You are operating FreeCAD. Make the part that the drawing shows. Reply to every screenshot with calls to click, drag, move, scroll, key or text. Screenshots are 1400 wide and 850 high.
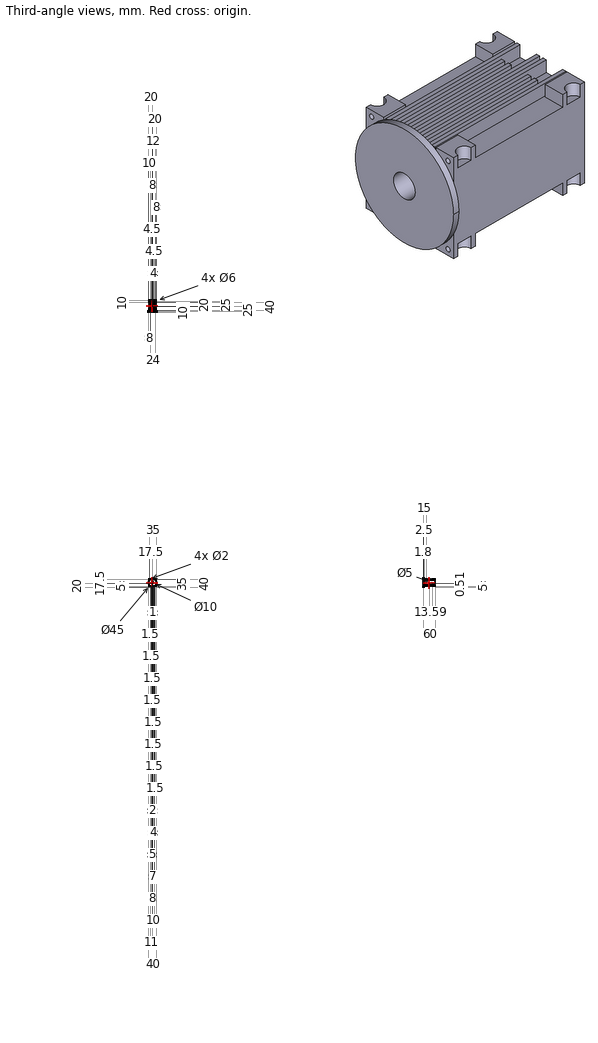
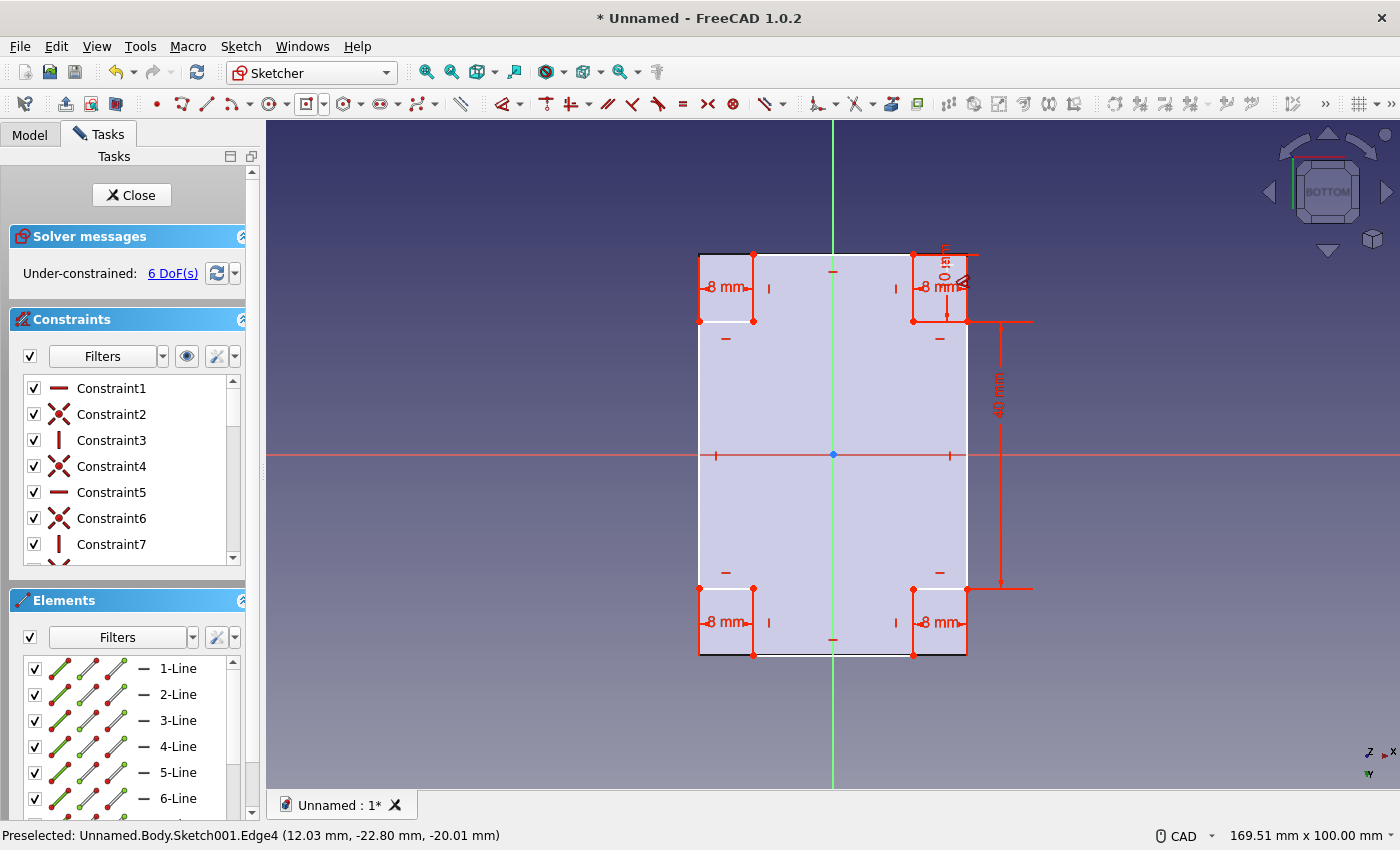
click(865, 255)
click(796, 221)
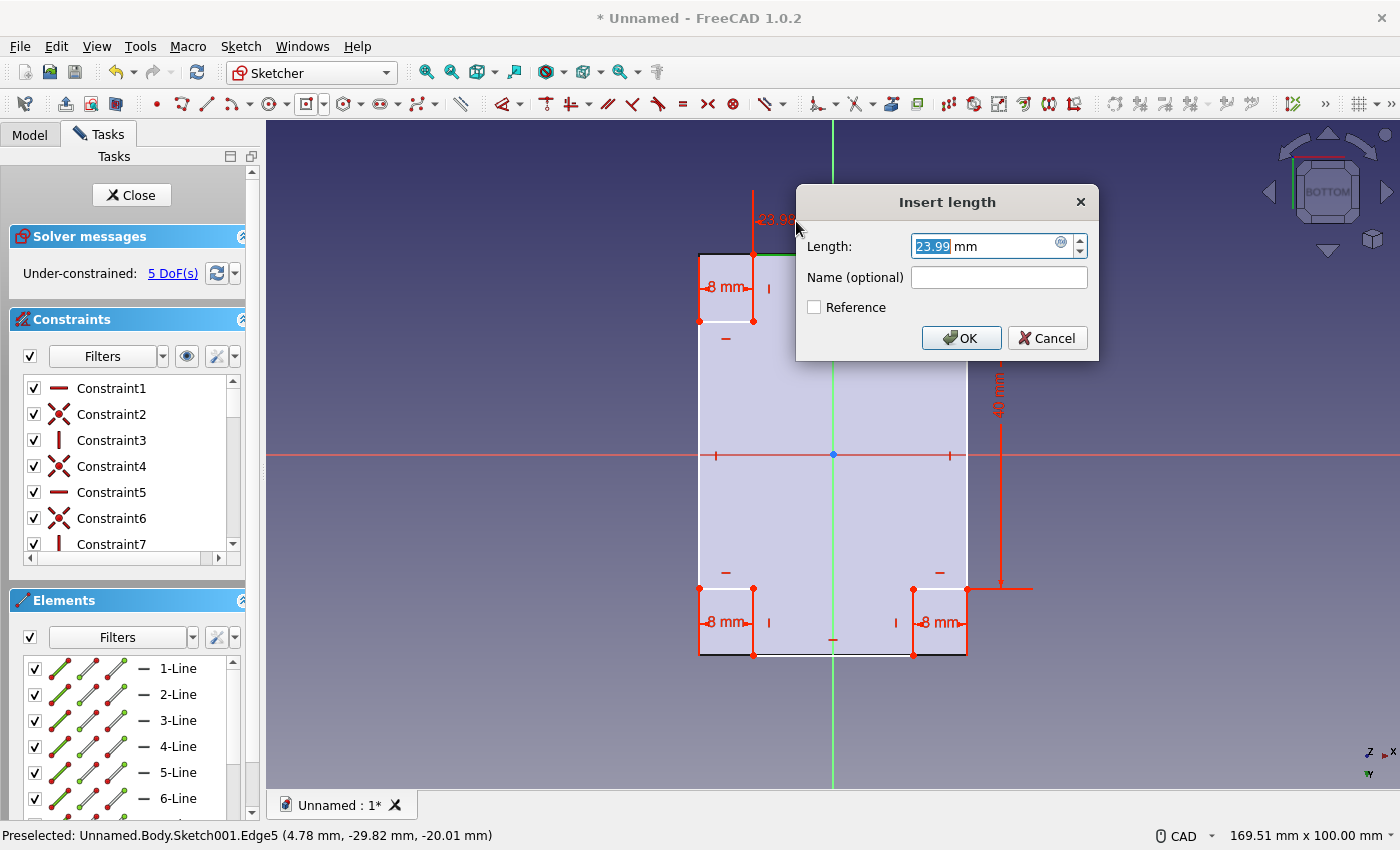
text(24)
key(Return)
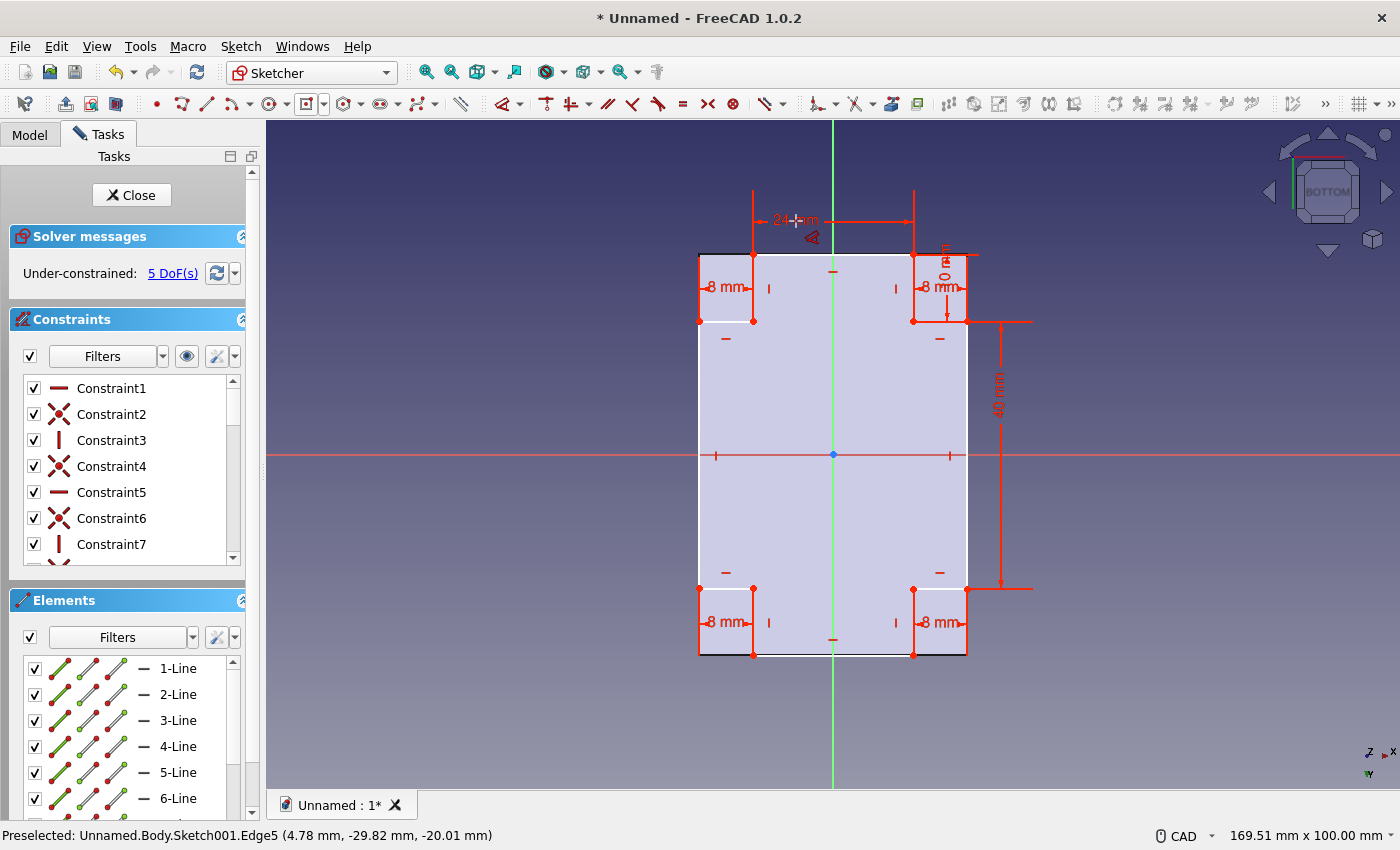
click(753, 275)
click(719, 265)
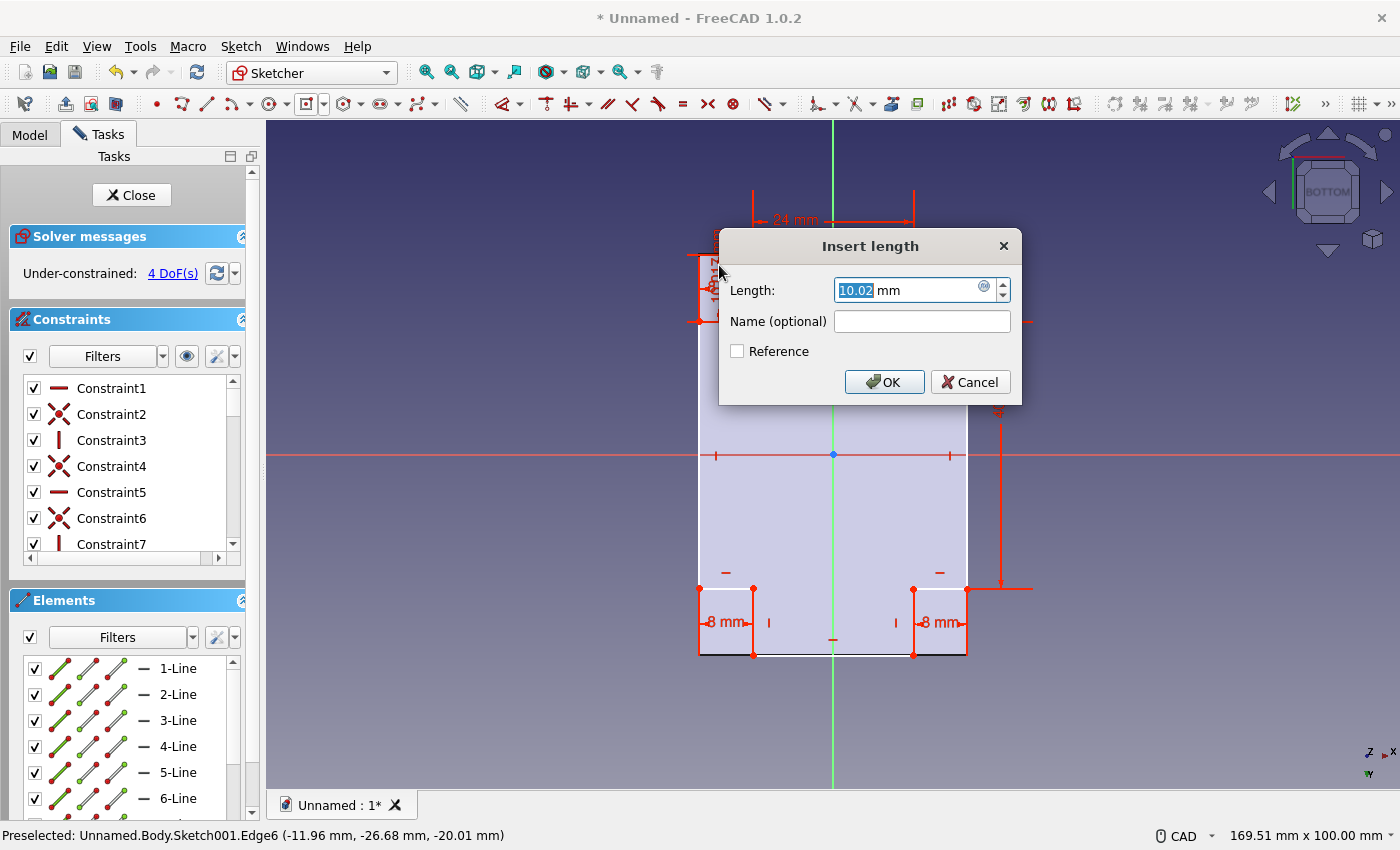
text(10)
key(Return)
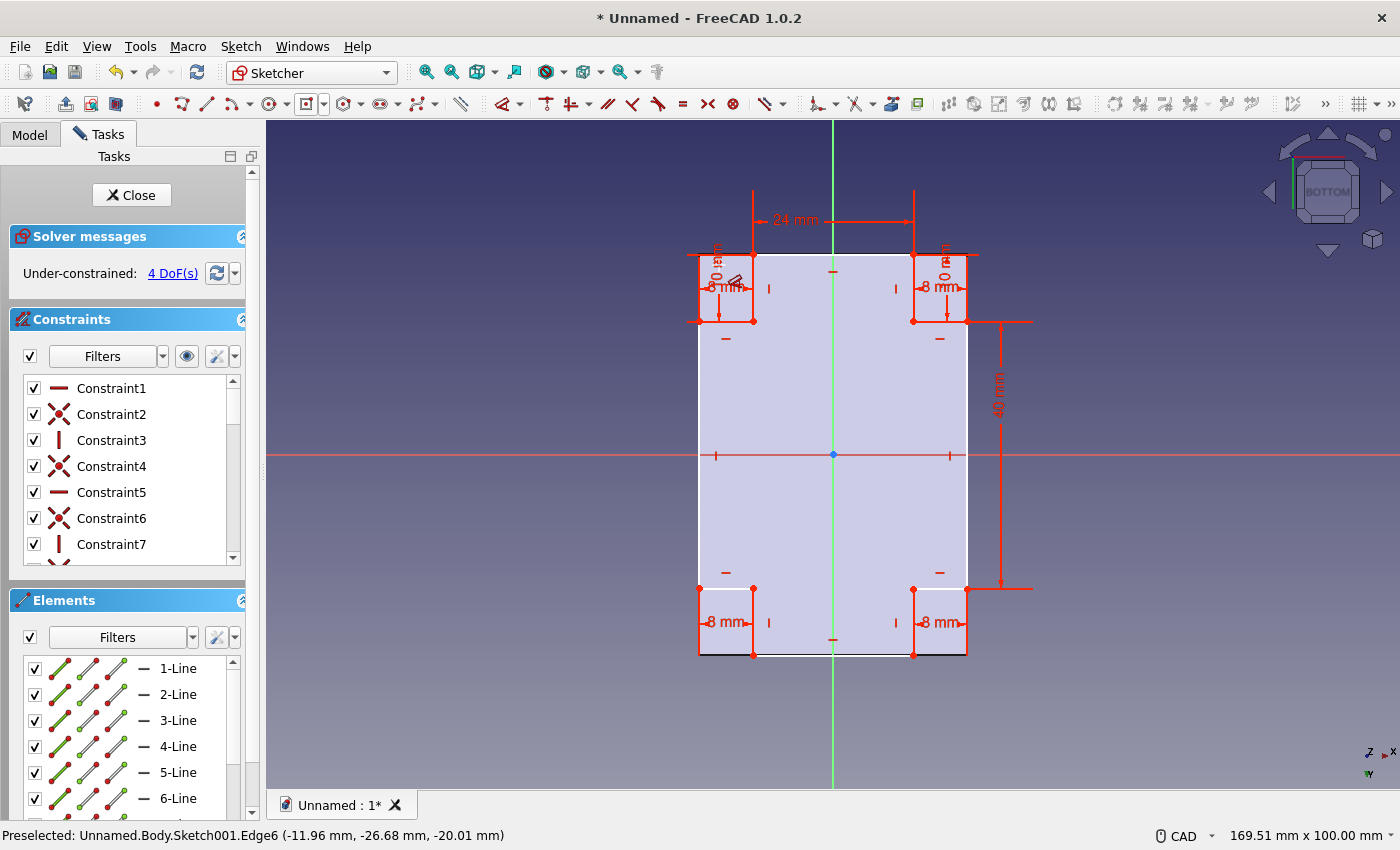
click(699, 402)
click(665, 394)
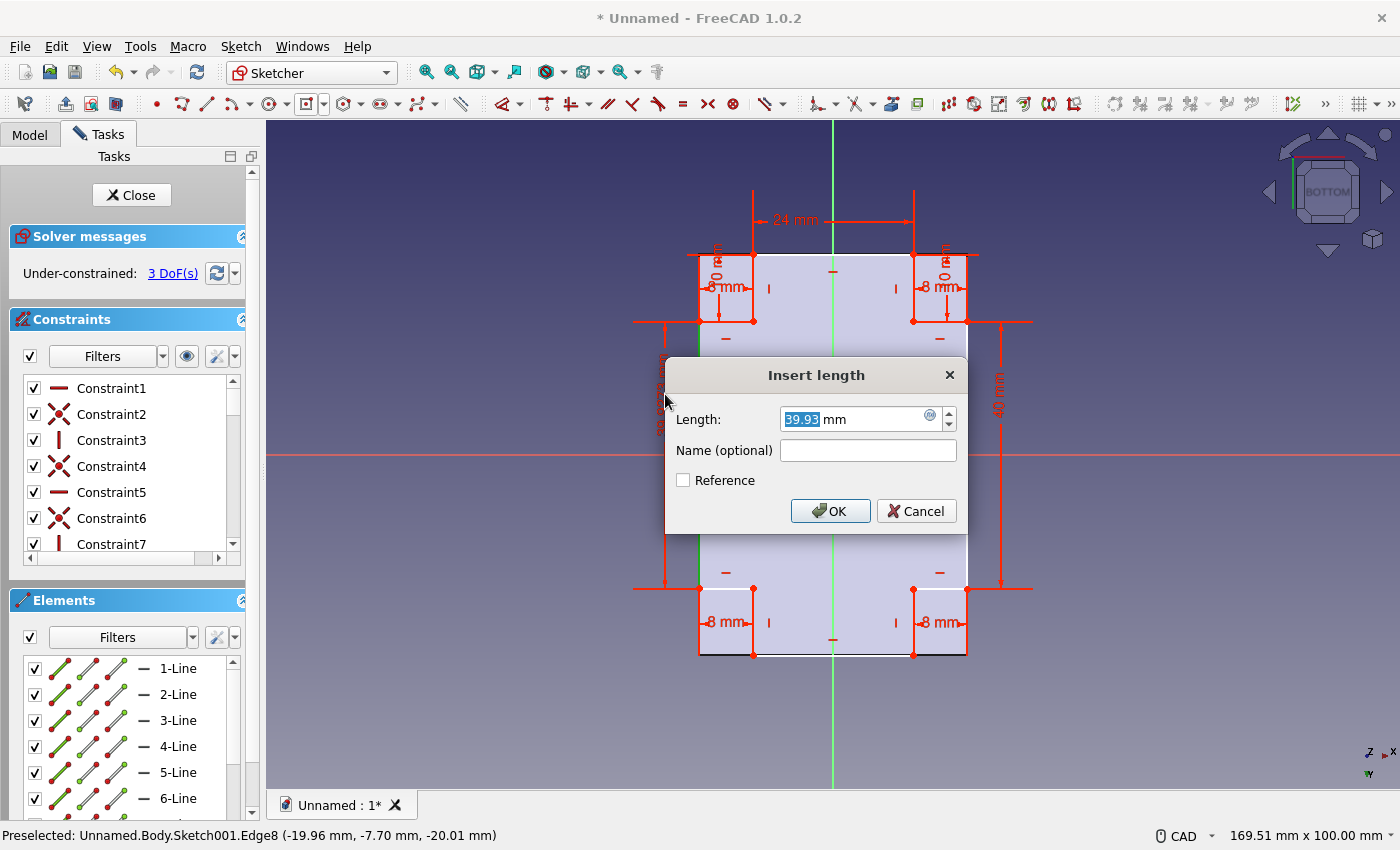
text(40)
key(Return)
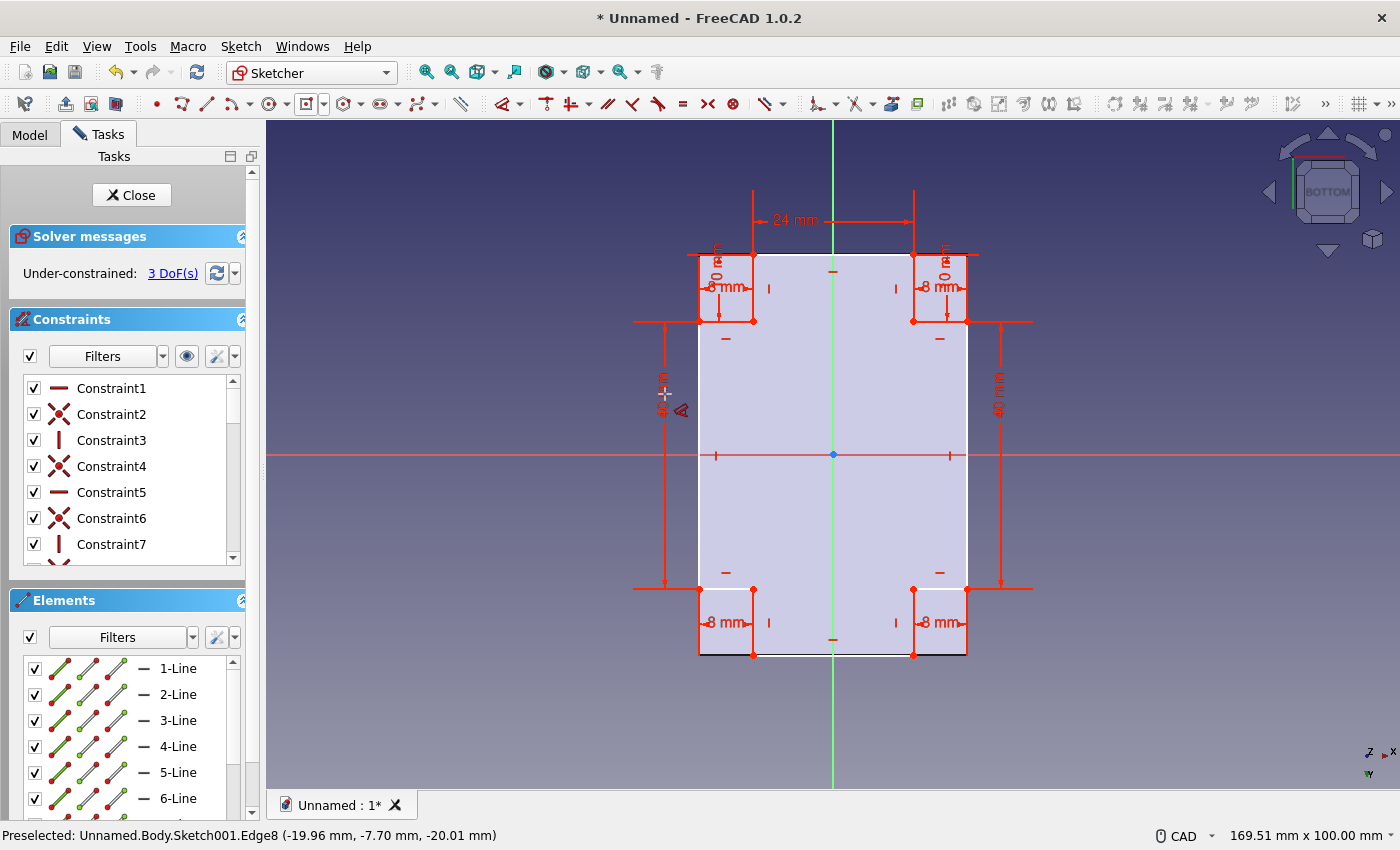
click(753, 609)
click(719, 646)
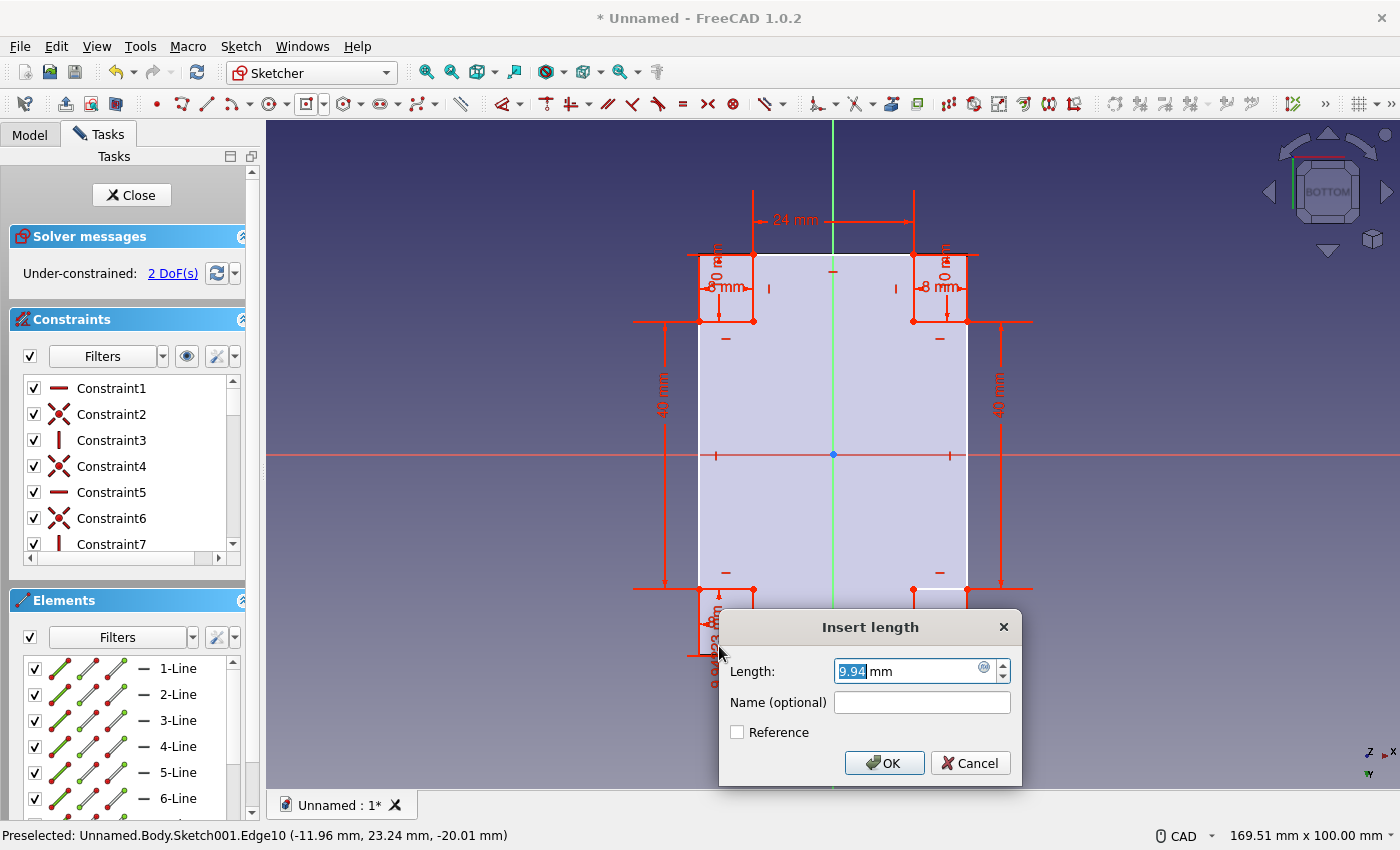
text(10)
key(Return)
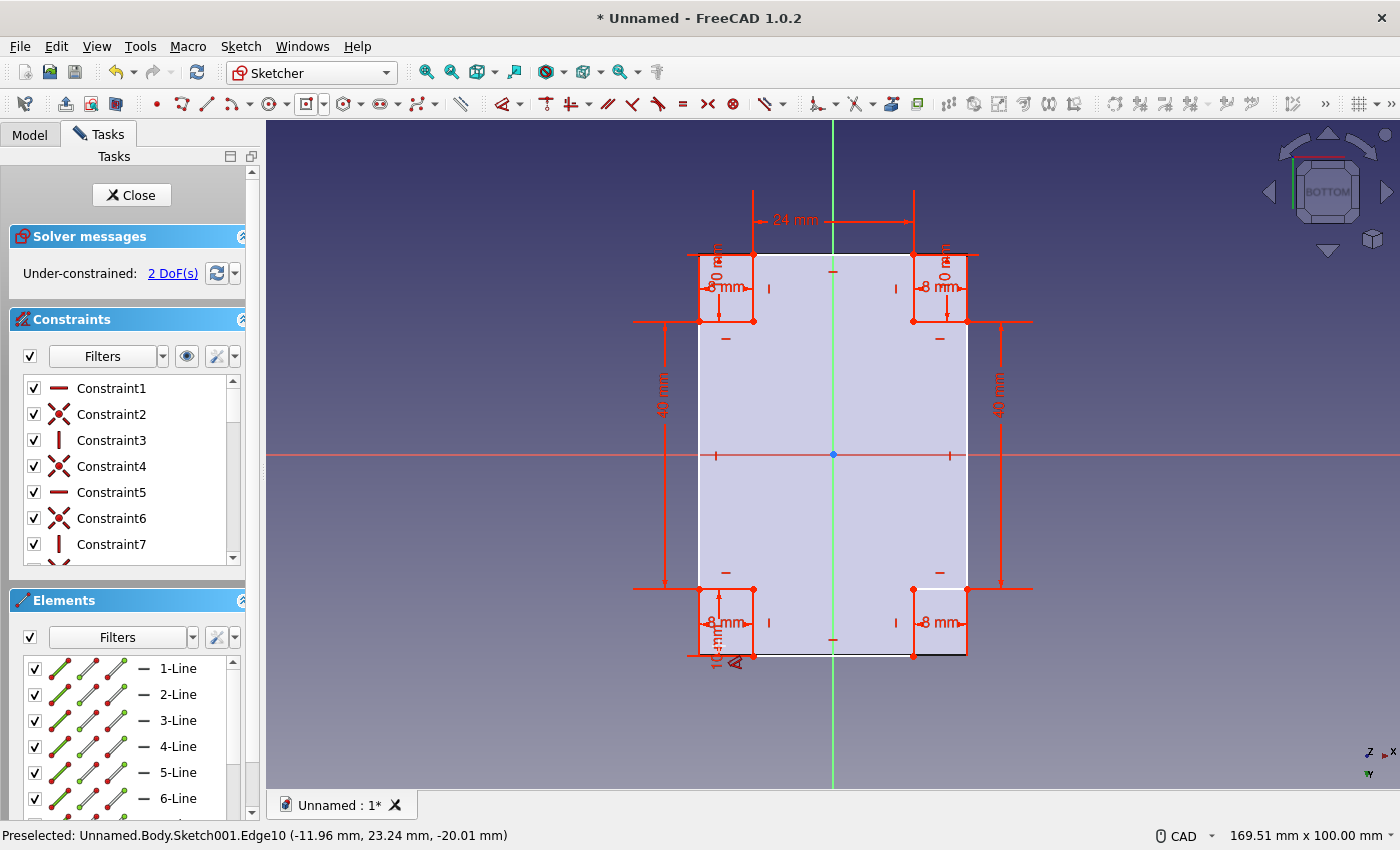
click(914, 589)
click(855, 623)